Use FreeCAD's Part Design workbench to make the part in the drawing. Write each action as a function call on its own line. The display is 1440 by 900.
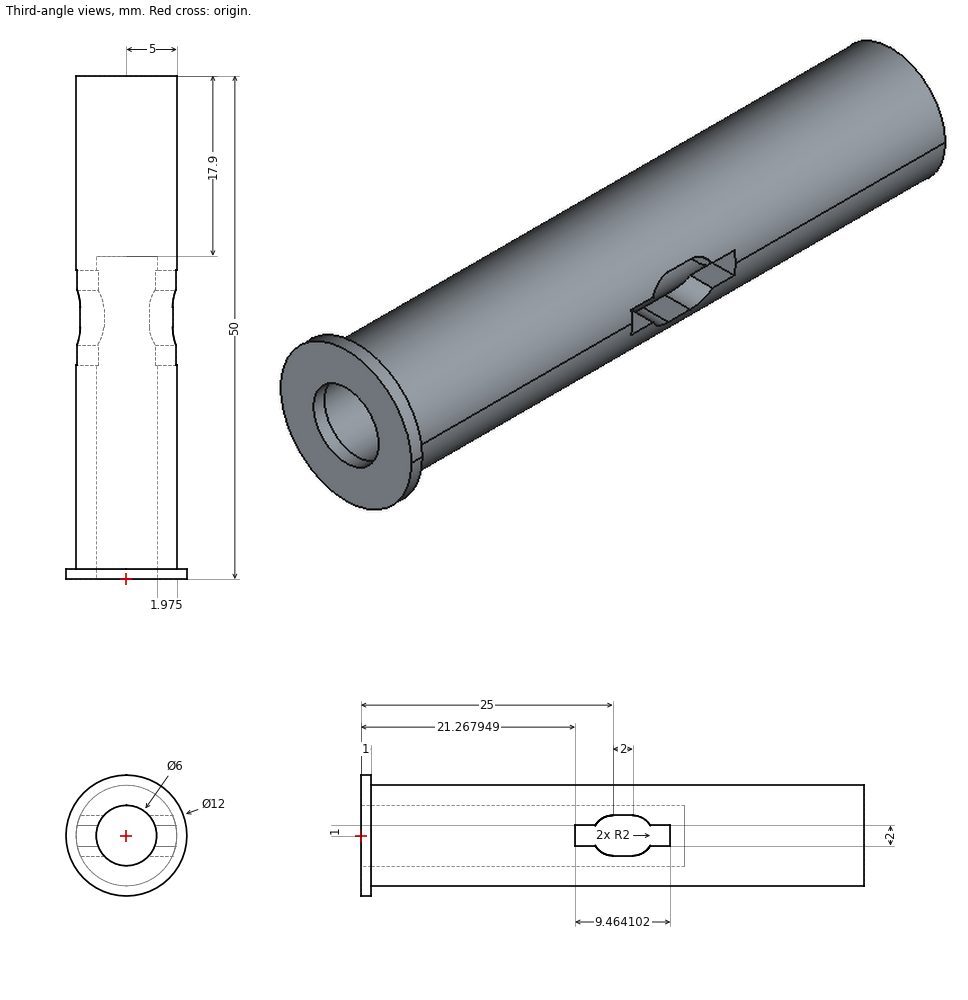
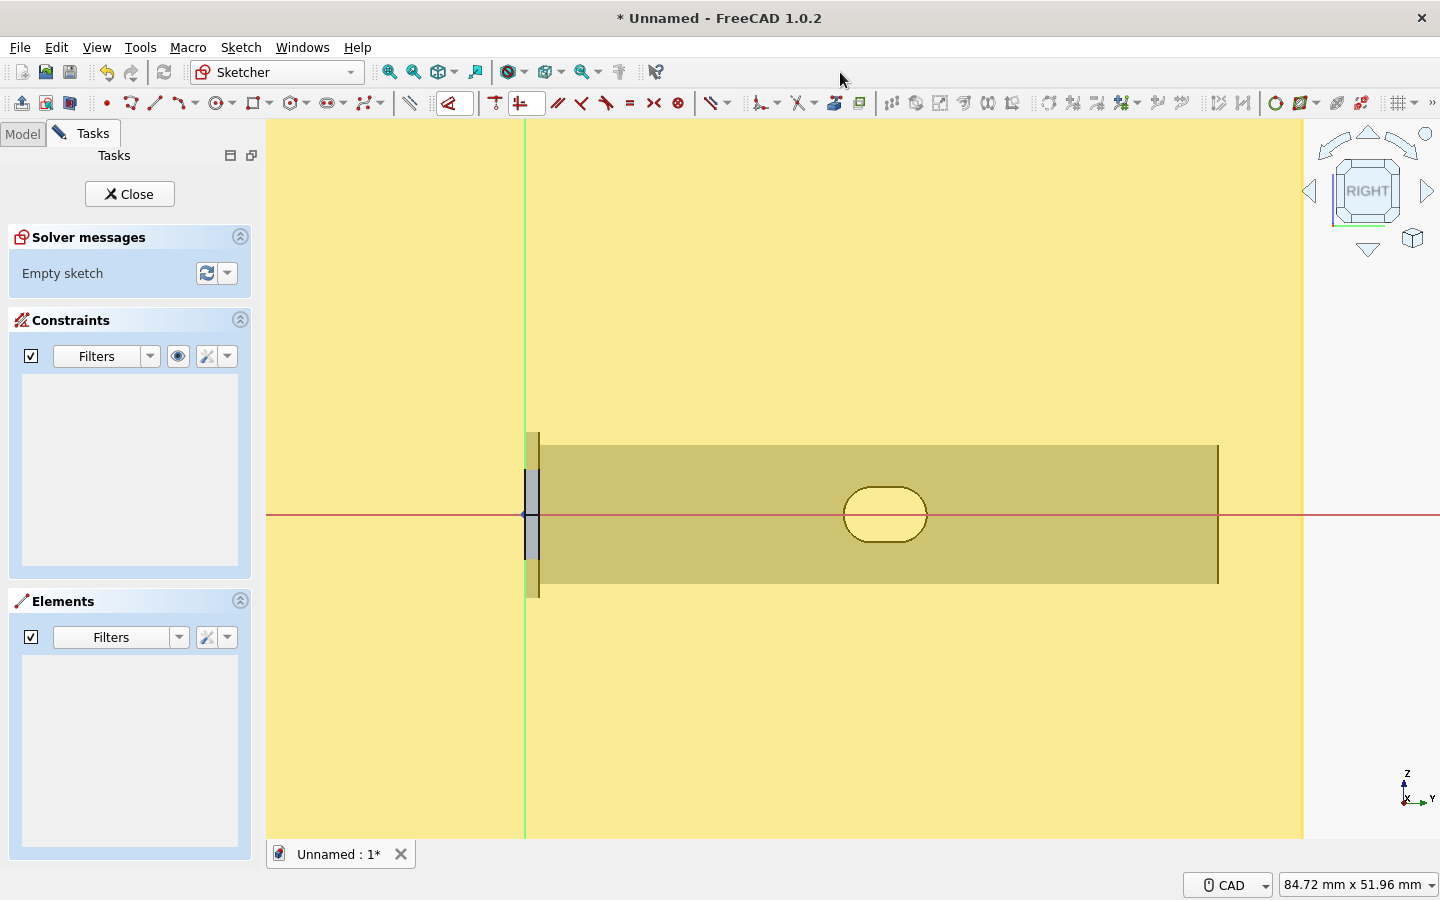
key(q)
key(s)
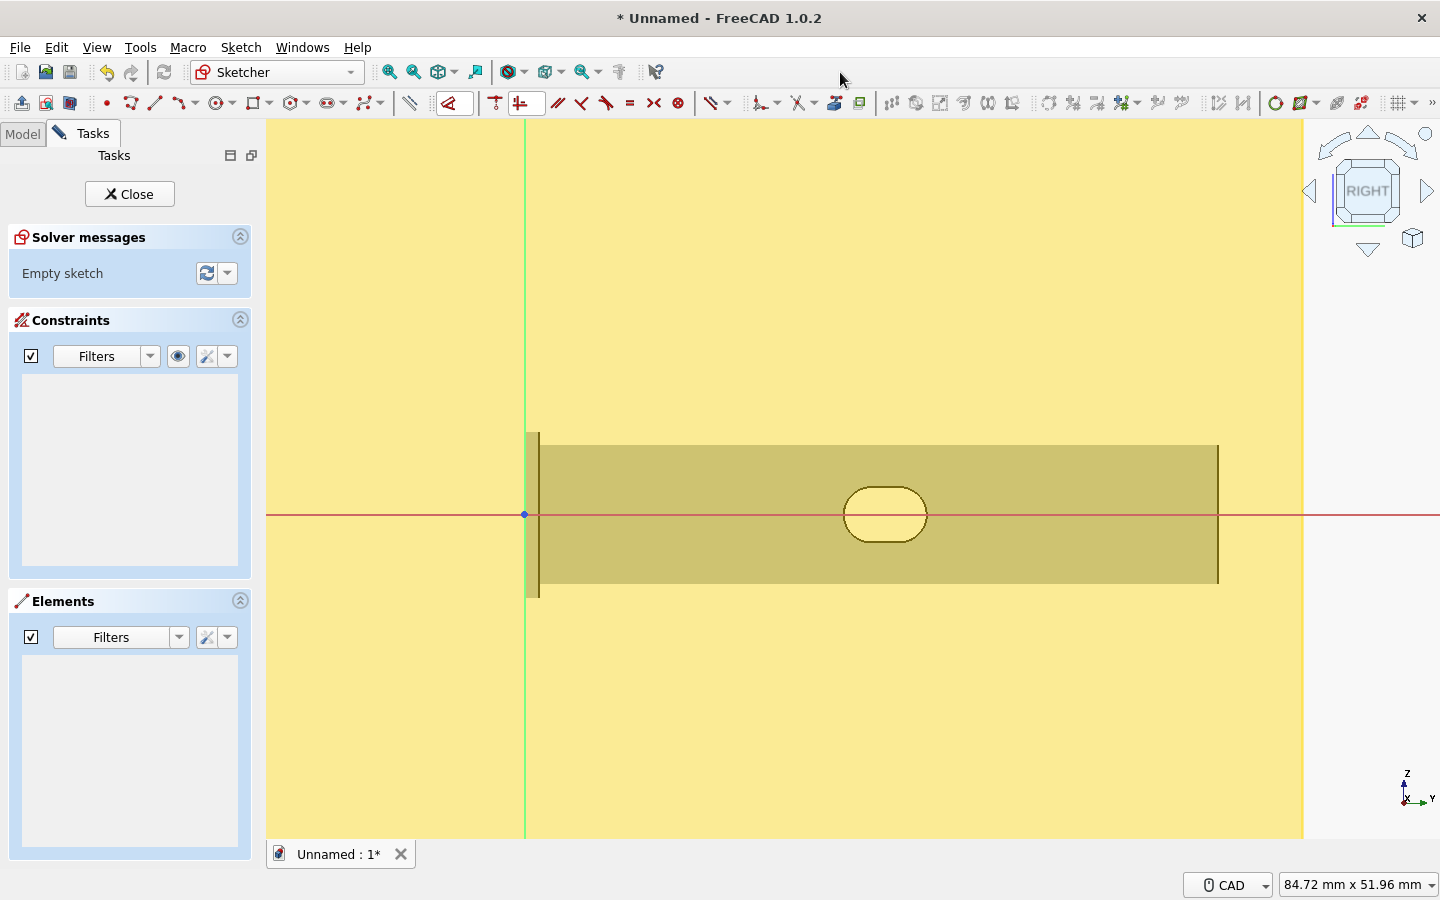
scroll(911, 524, up, 8)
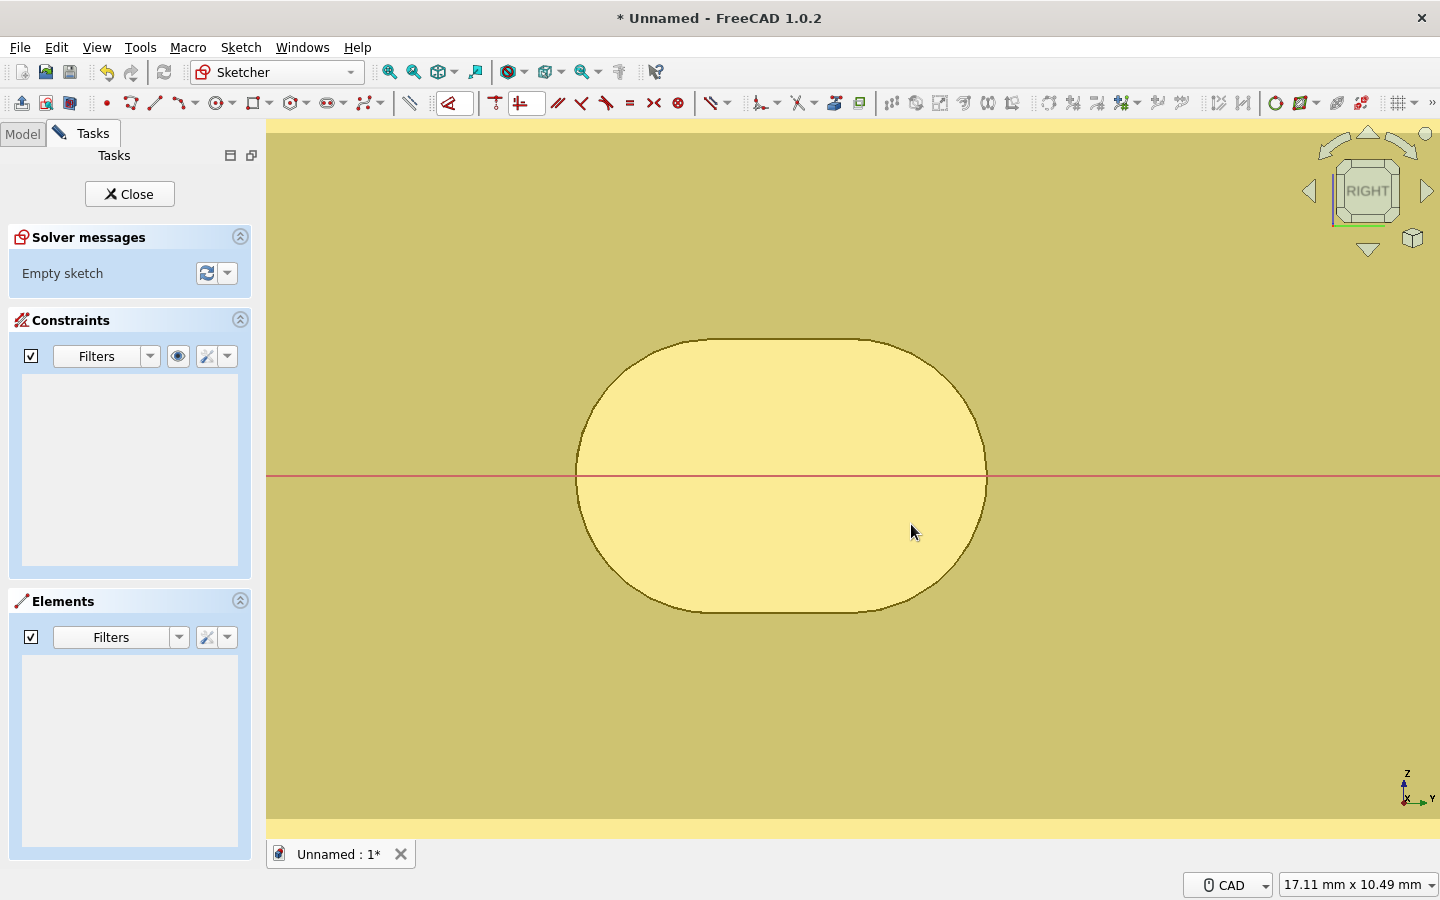
click(254, 104)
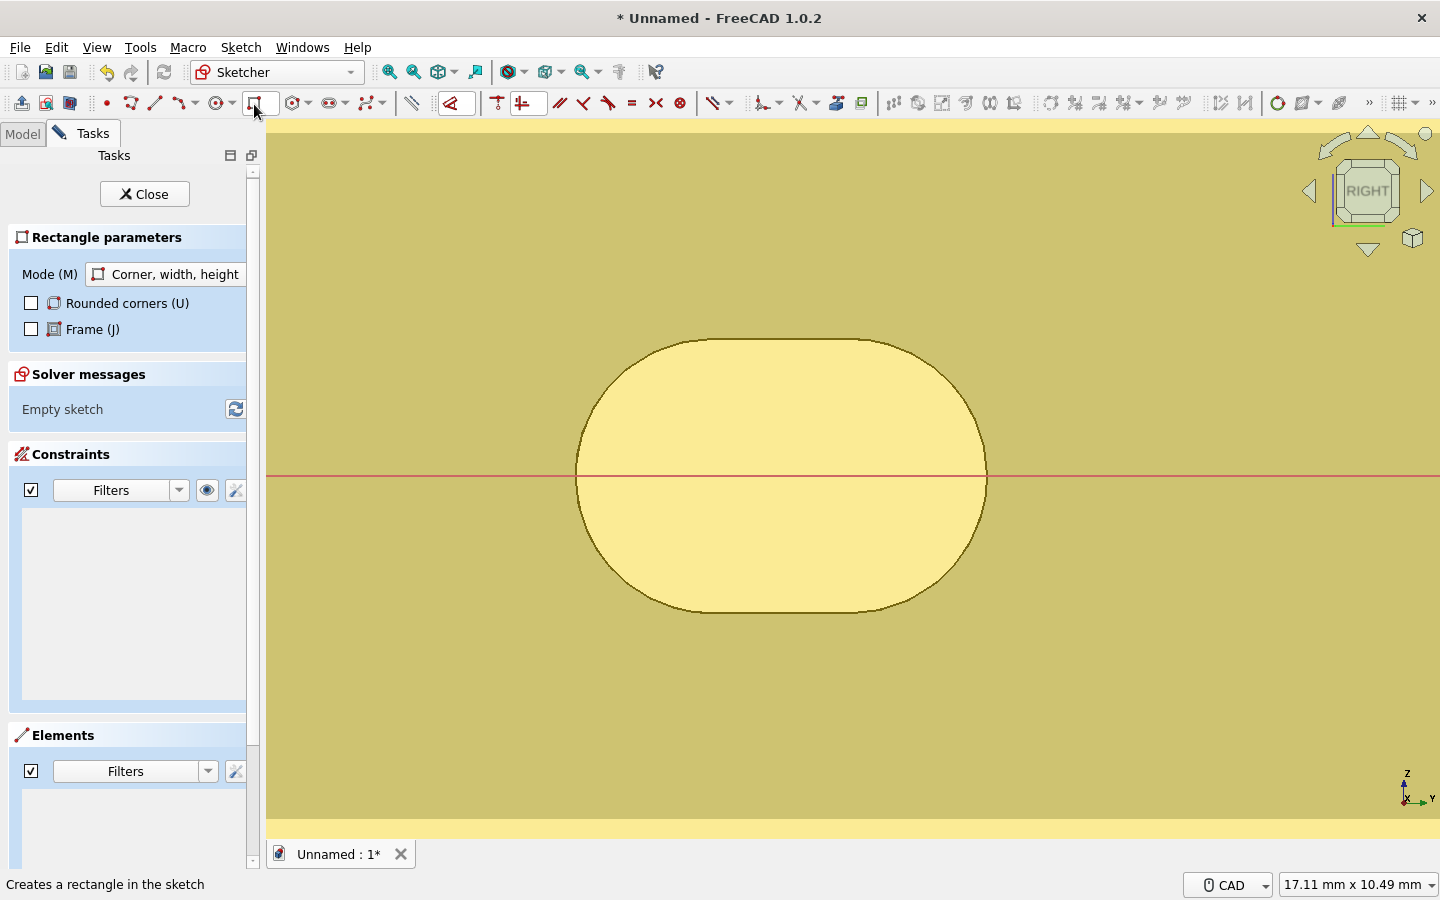
click(457, 407)
move(1106, 545)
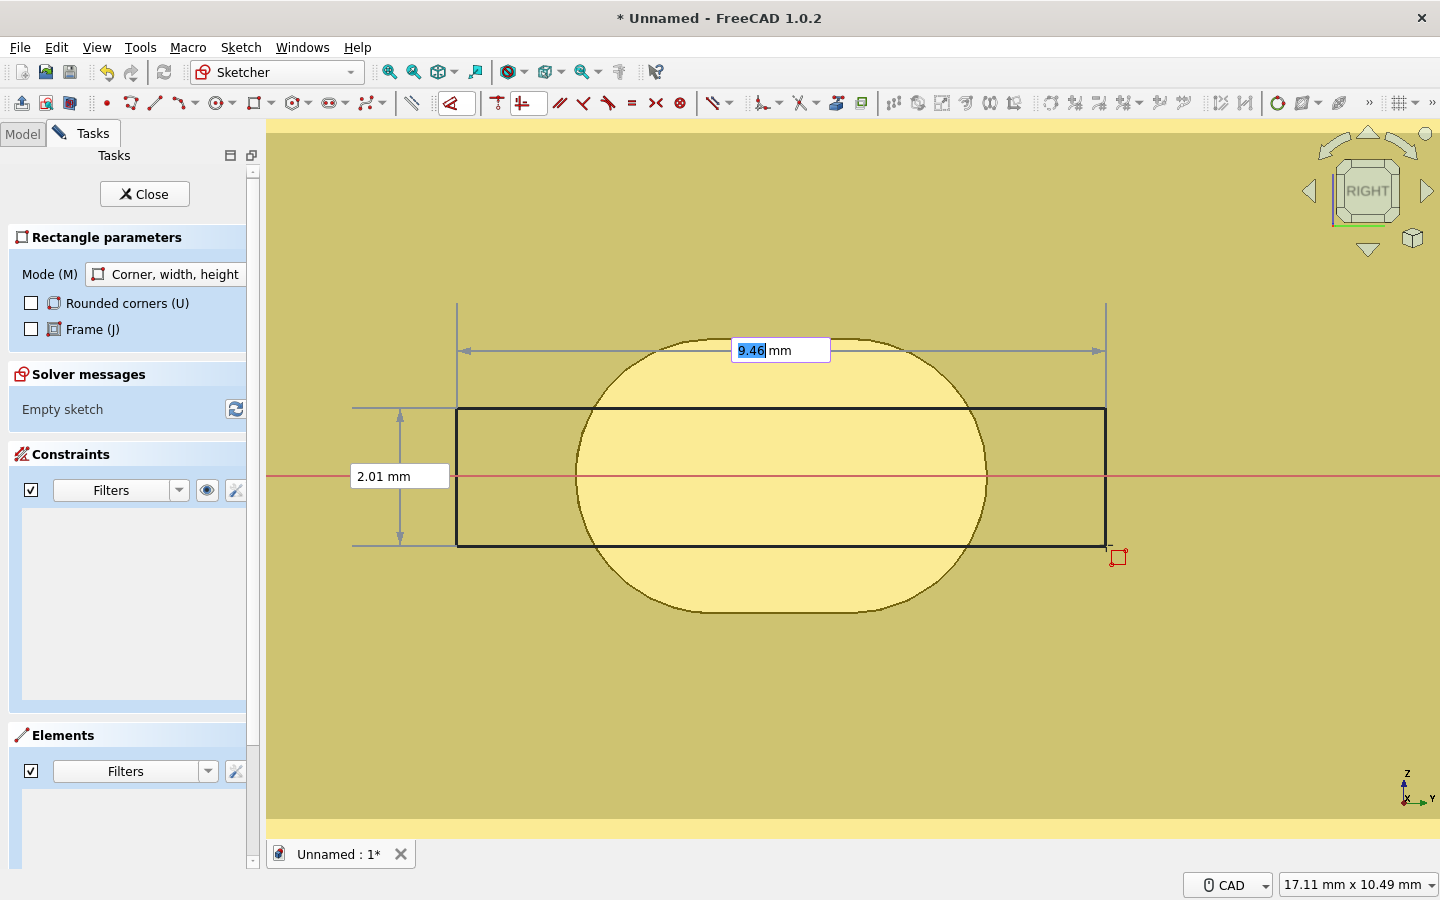
text(9.464102)
key(Tab)
text(2)
key(Return)
key(Escape)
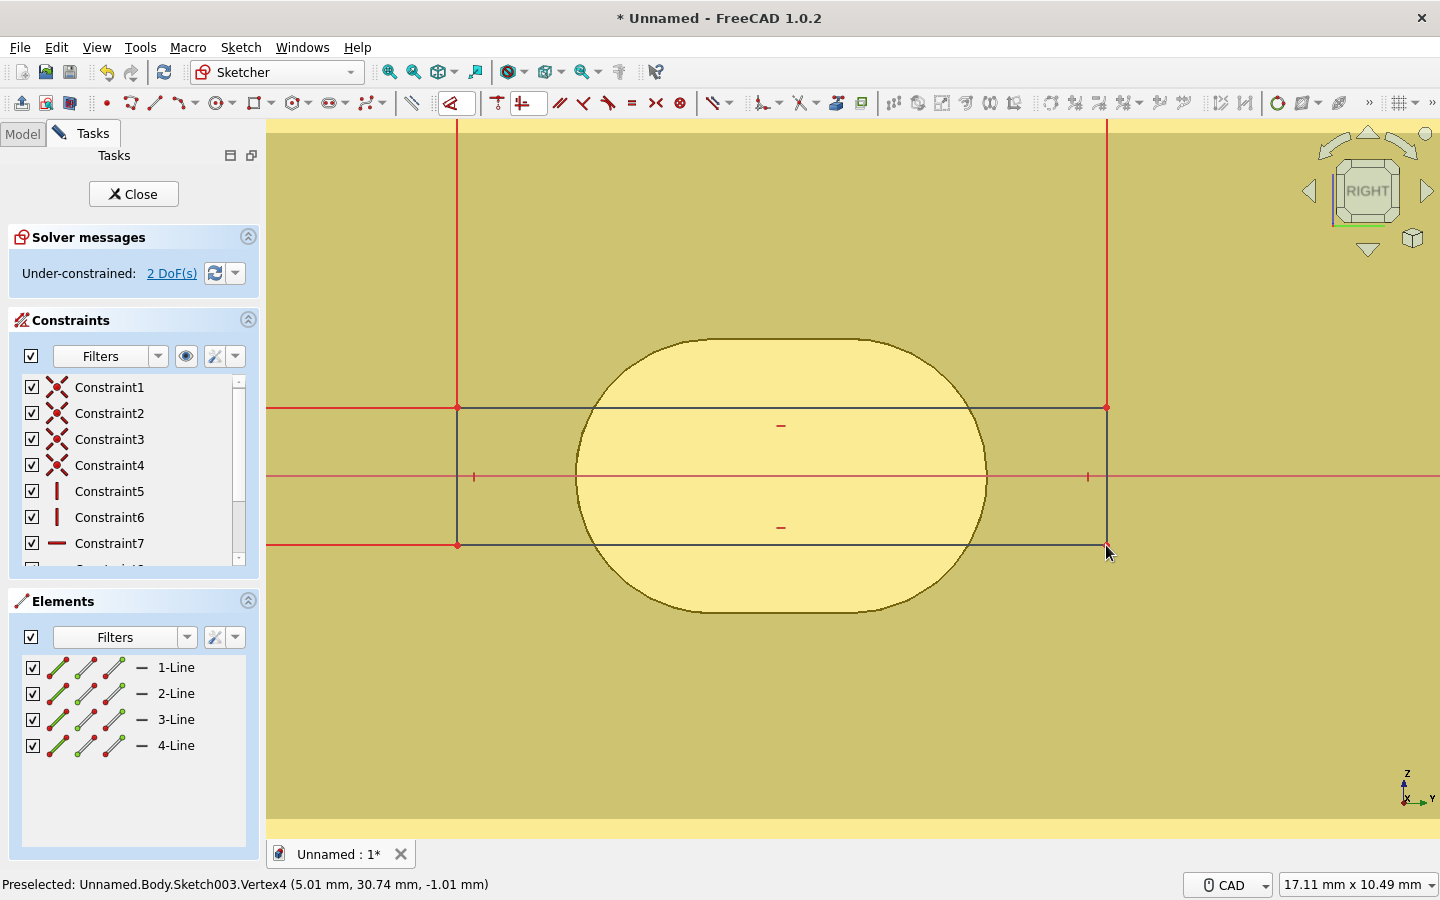
click(457, 408)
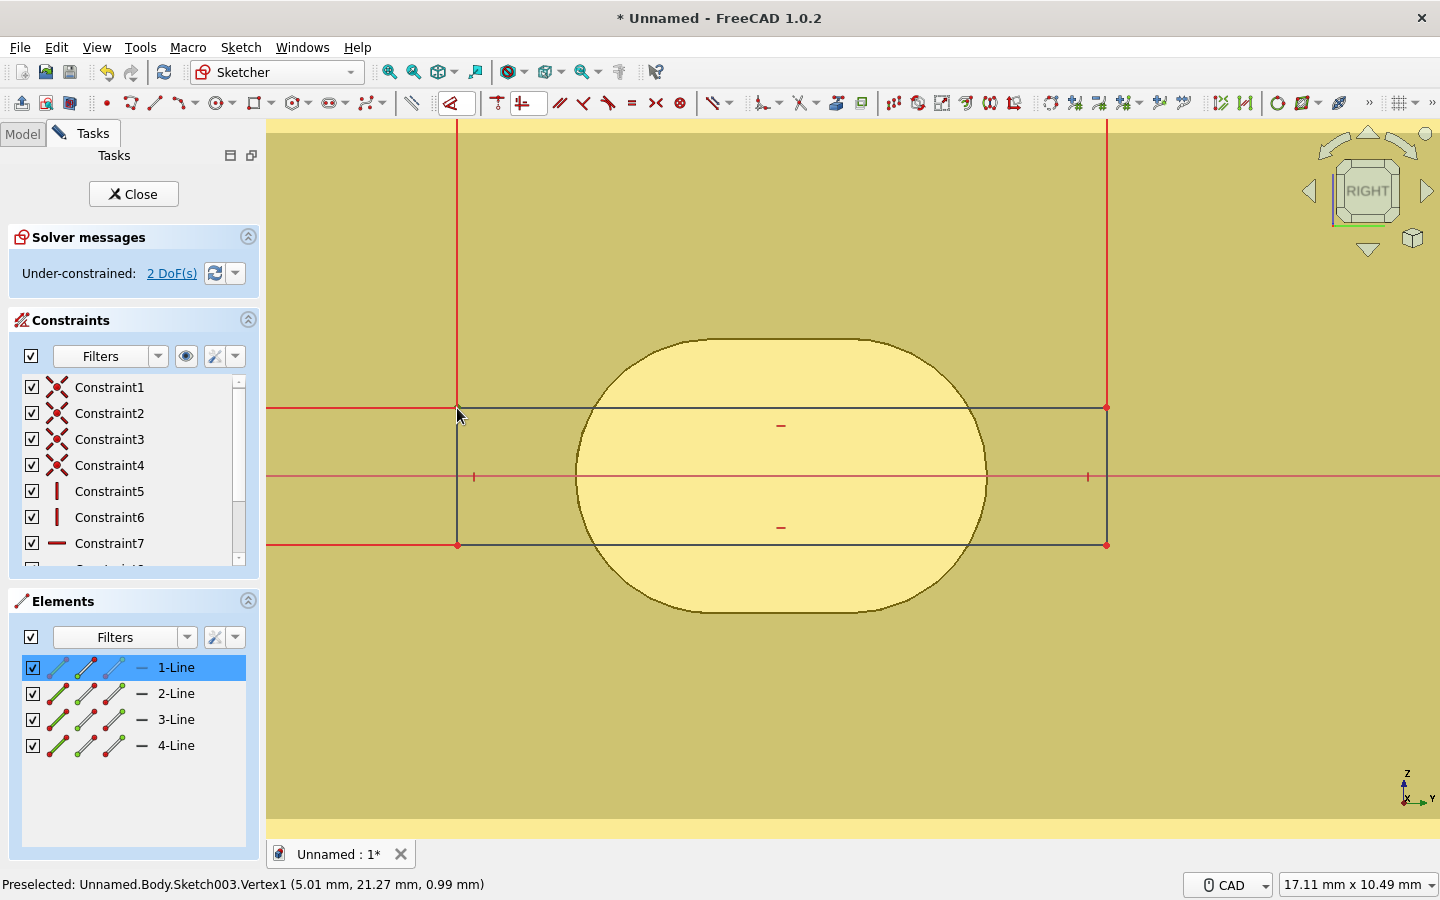
key(i)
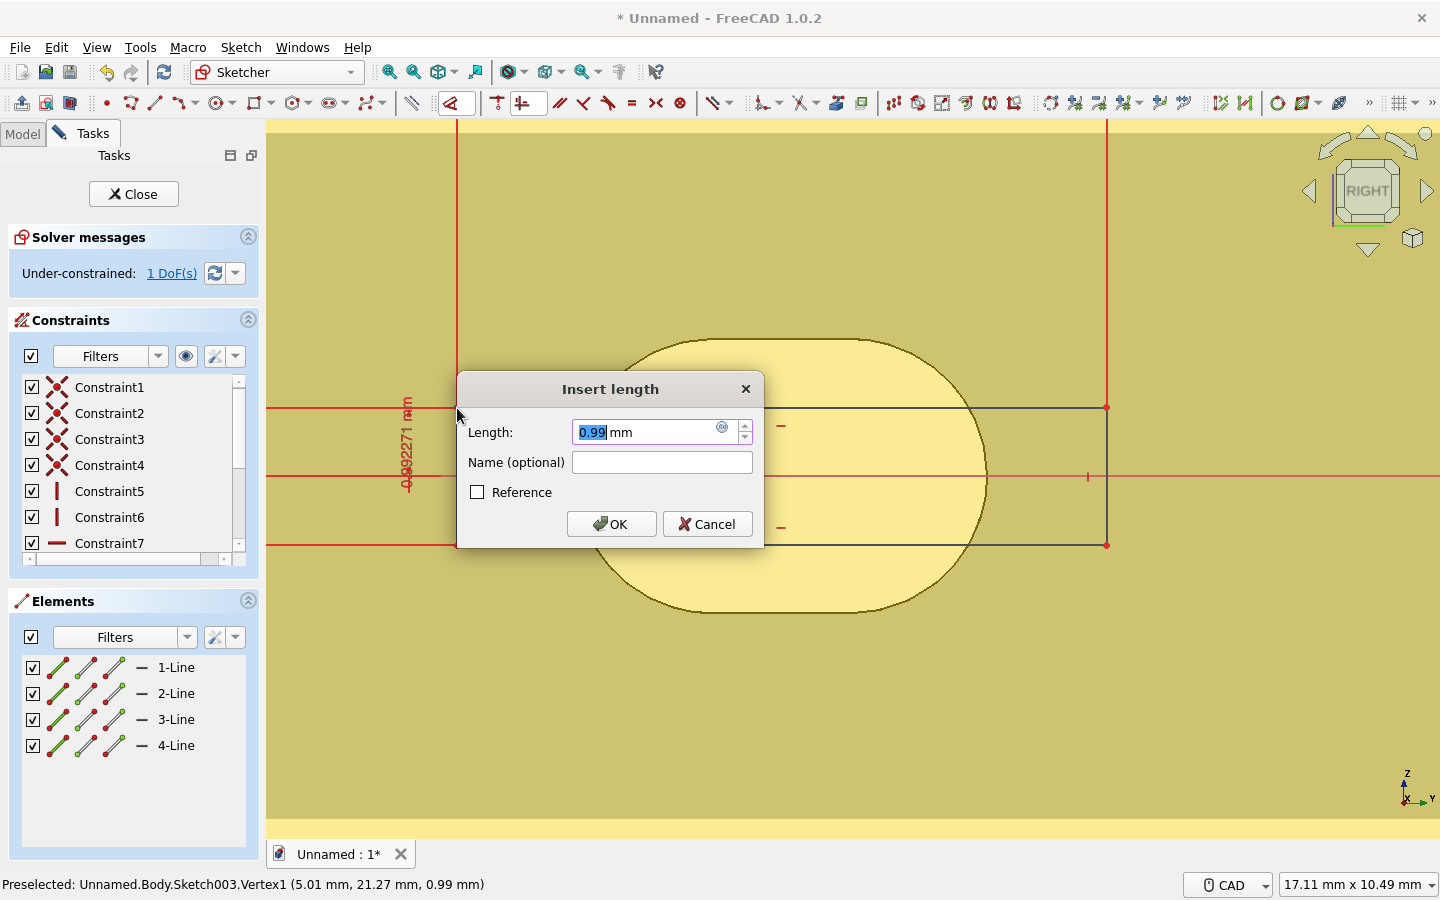
text(1)
key(Return)